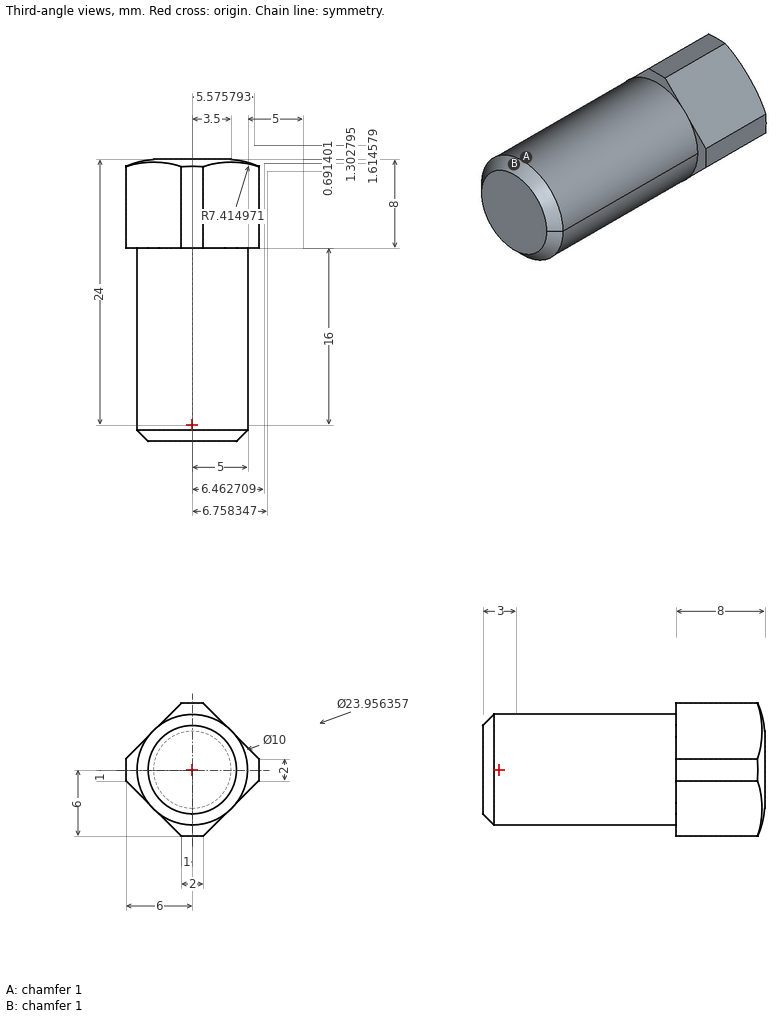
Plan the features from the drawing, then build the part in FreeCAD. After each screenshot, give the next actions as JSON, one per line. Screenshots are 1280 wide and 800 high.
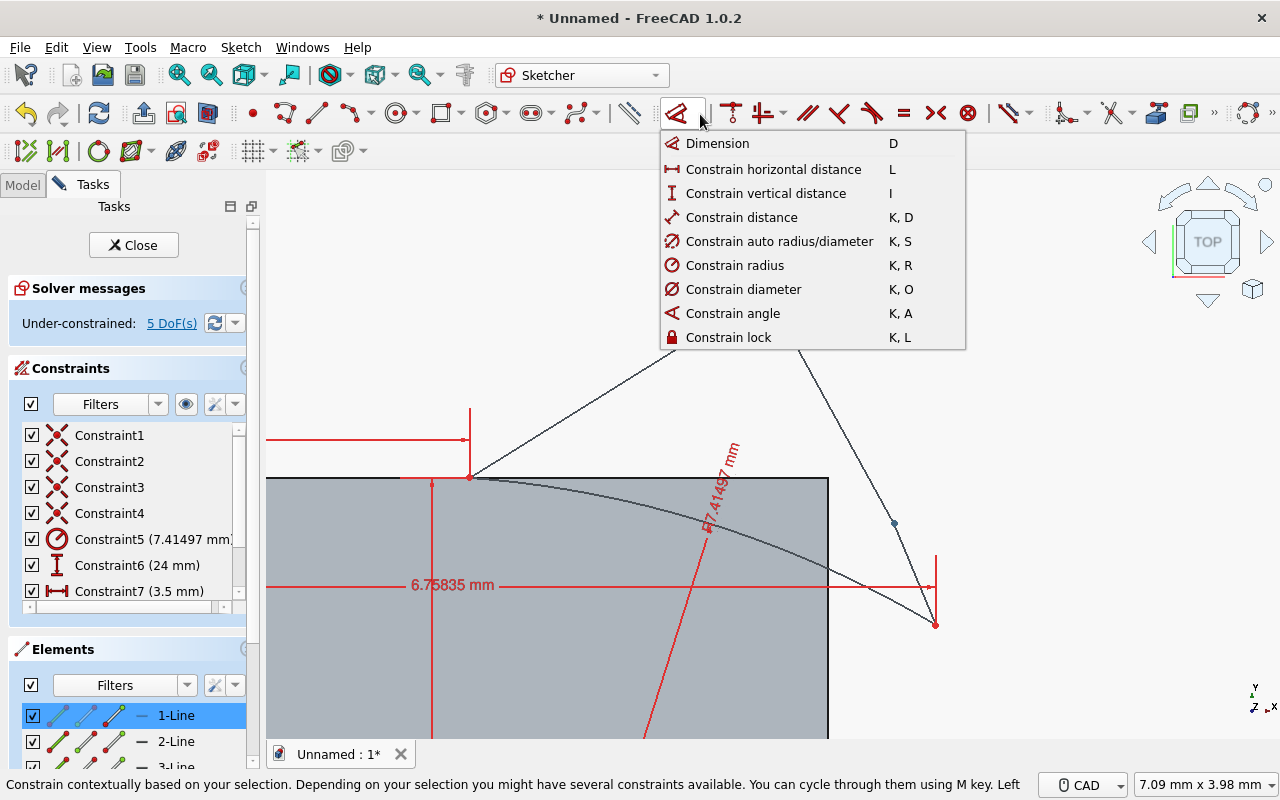
{"action": "left_click", "coordinate": [813, 169]}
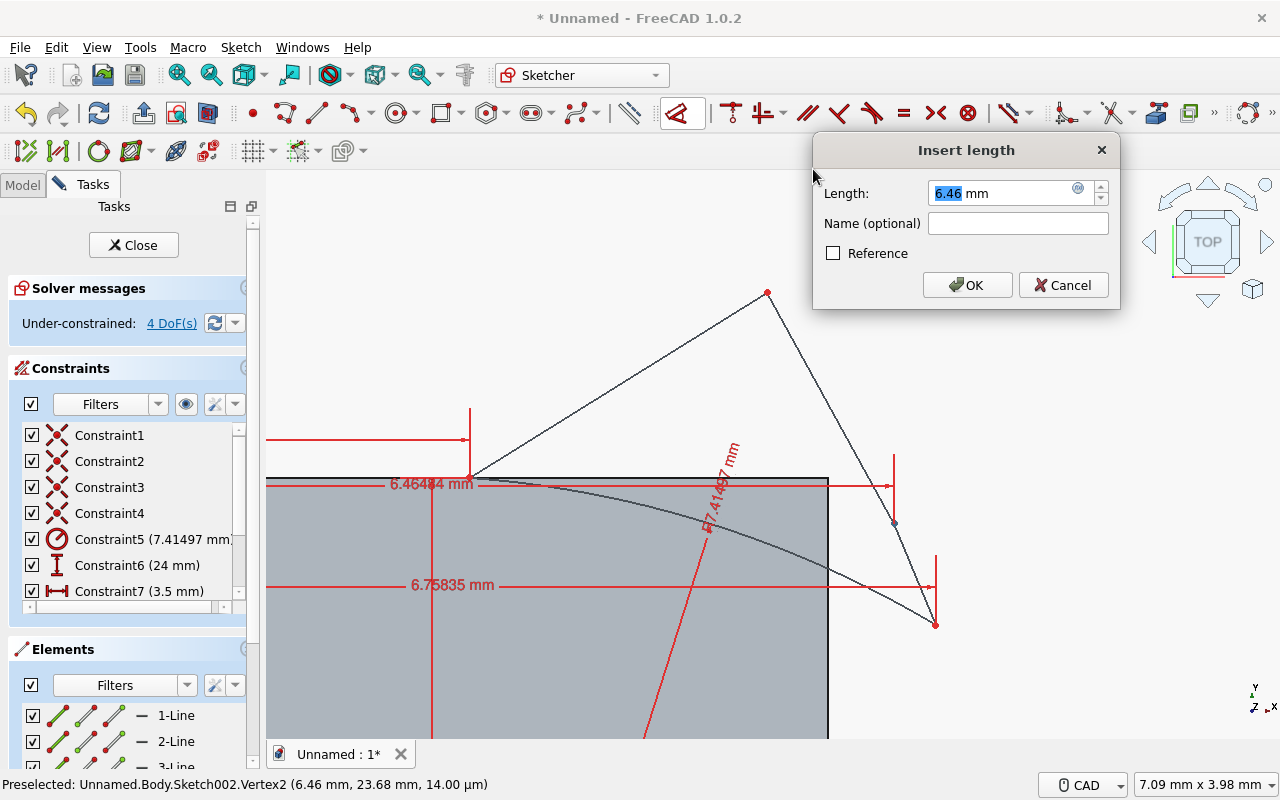
{"action": "type", "text": "6.462709"}
{"action": "key", "text": "Return"}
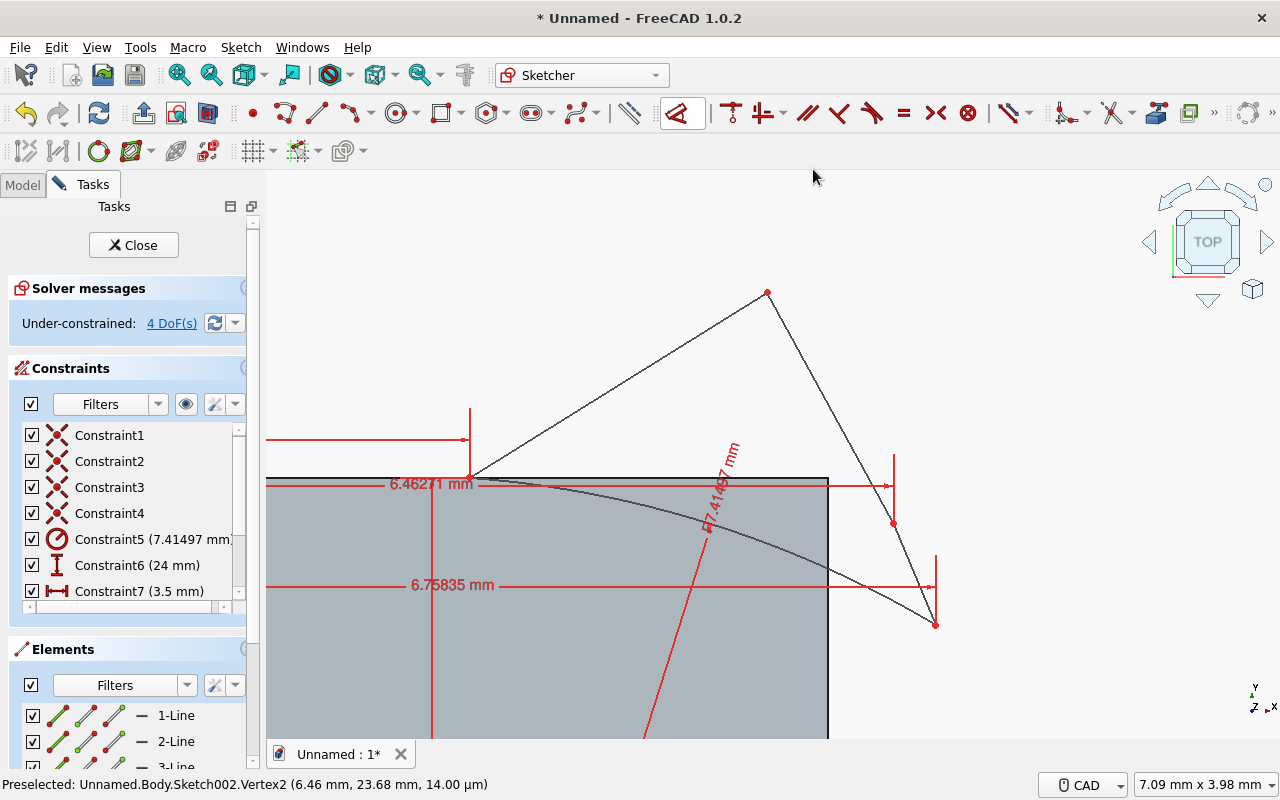
{"action": "left_click", "coordinate": [767, 293]}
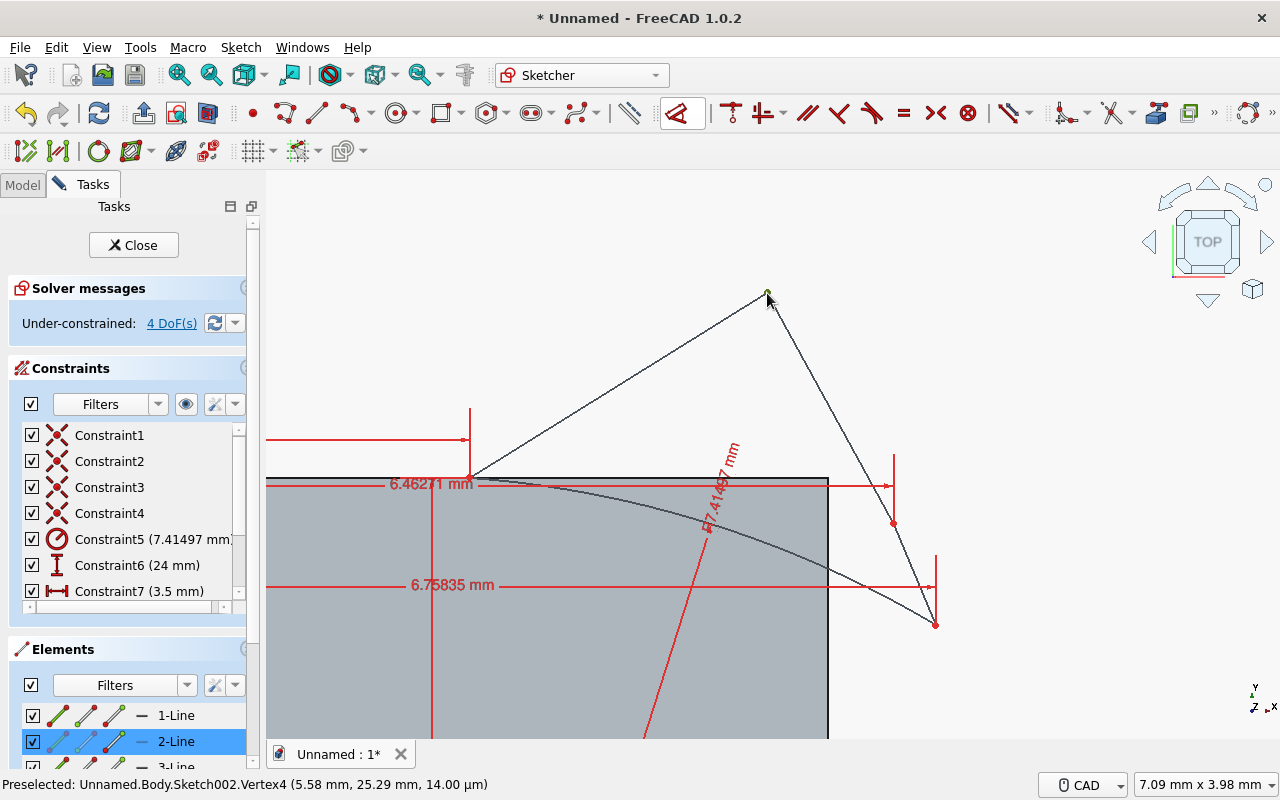
{"action": "left_click", "coordinate": [700, 114]}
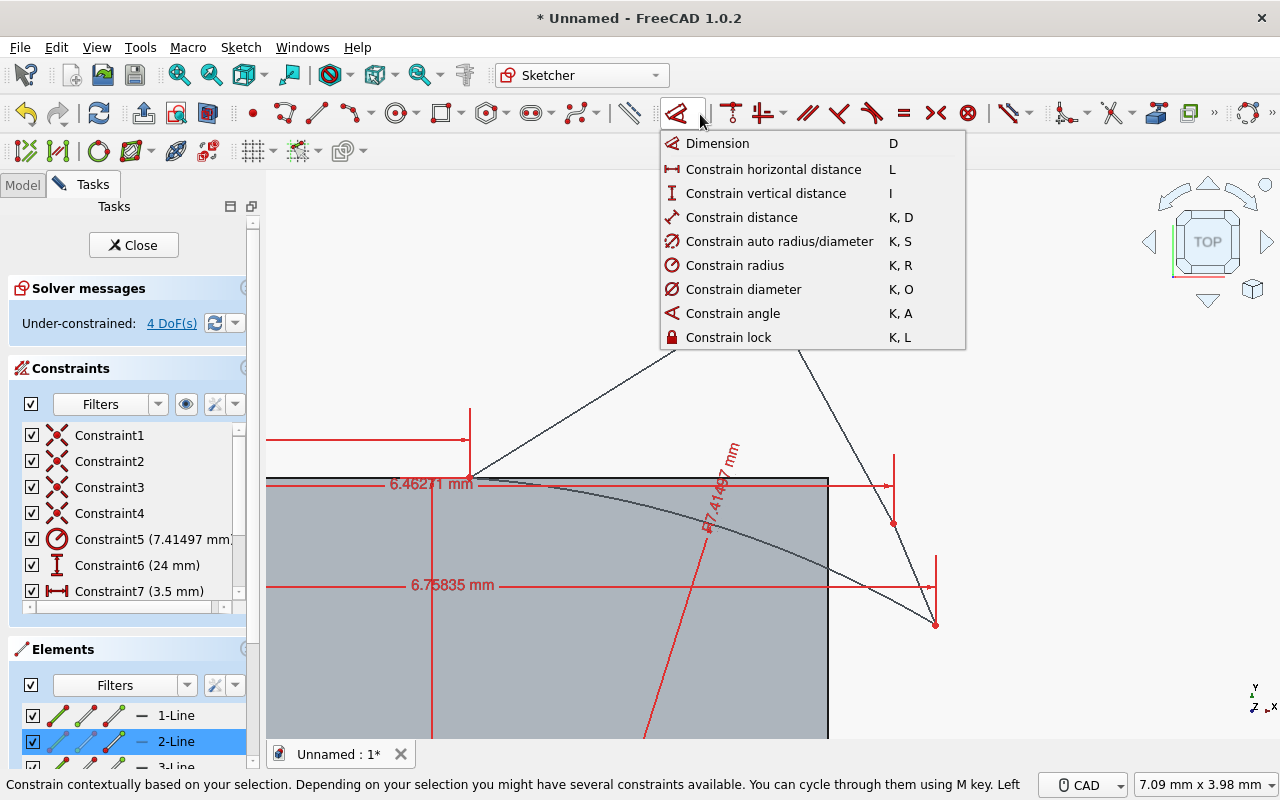
{"action": "left_click", "coordinate": [813, 169]}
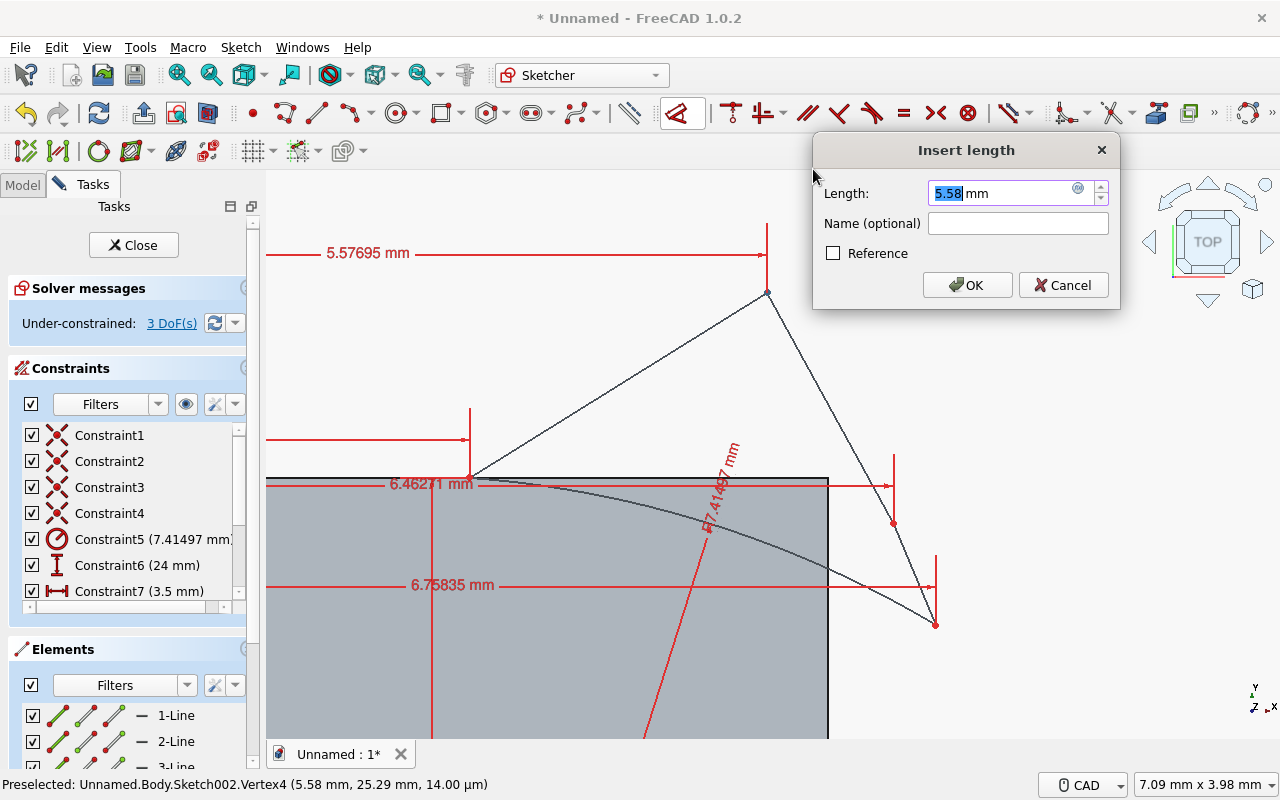
{"action": "type", "text": "5.575793"}
{"action": "key", "text": "Return"}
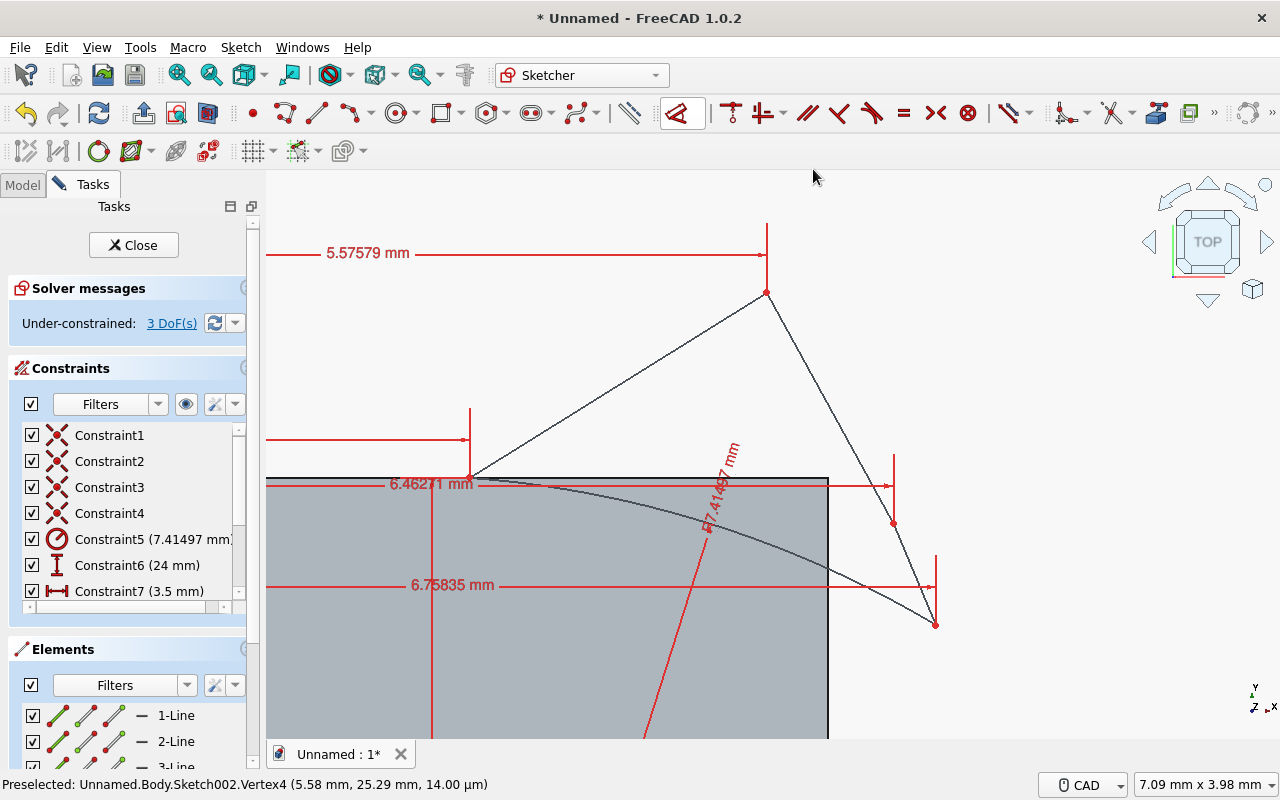
{"action": "left_click", "coordinate": [923, 595]}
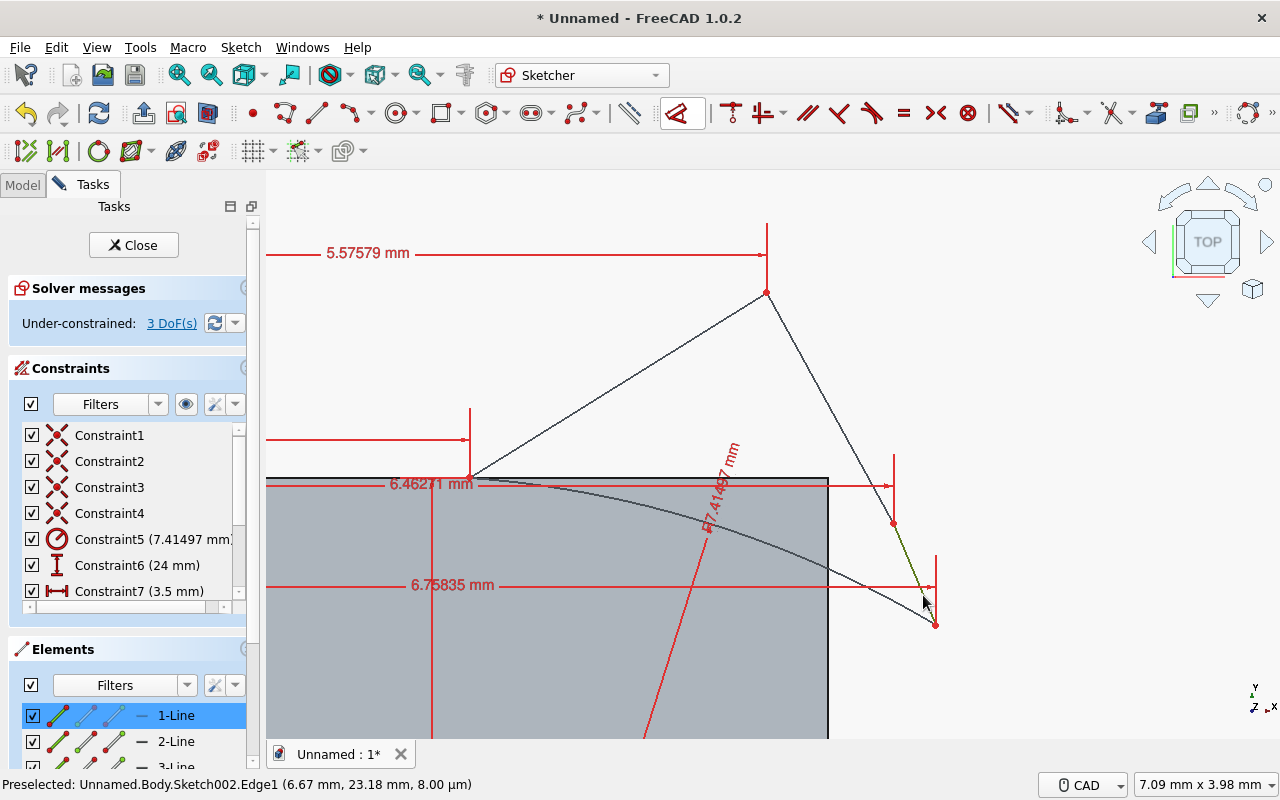
{"action": "left_click", "coordinate": [700, 114]}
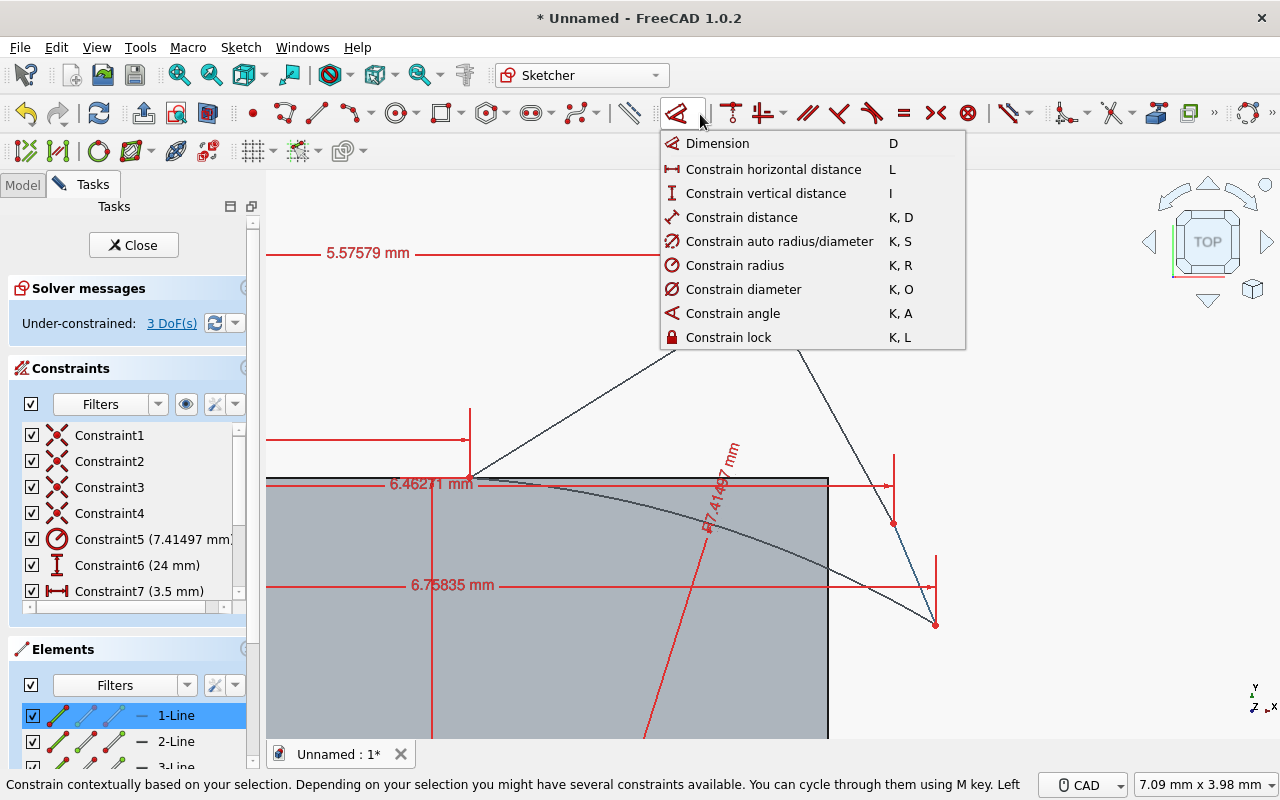
{"action": "left_click", "coordinate": [813, 193]}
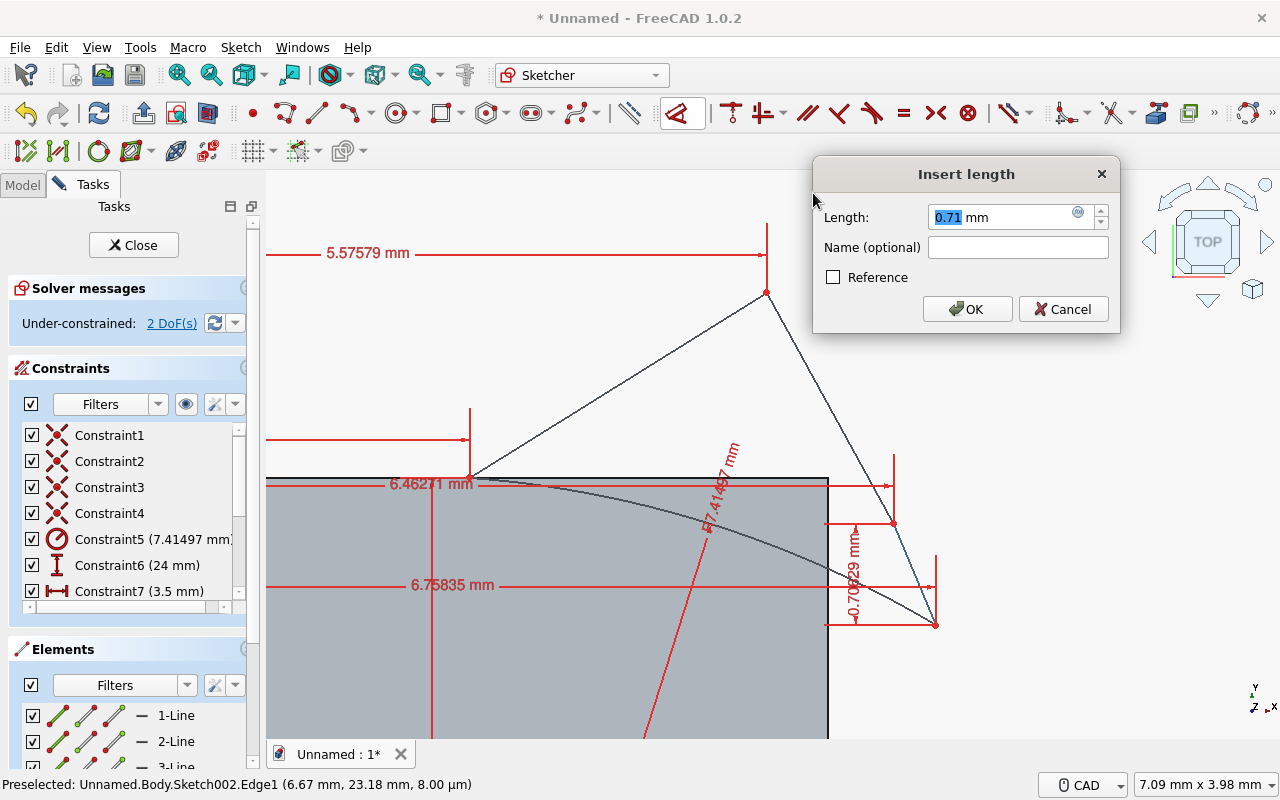
{"action": "type", "text": "0.691401"}
{"action": "key", "text": "Return"}